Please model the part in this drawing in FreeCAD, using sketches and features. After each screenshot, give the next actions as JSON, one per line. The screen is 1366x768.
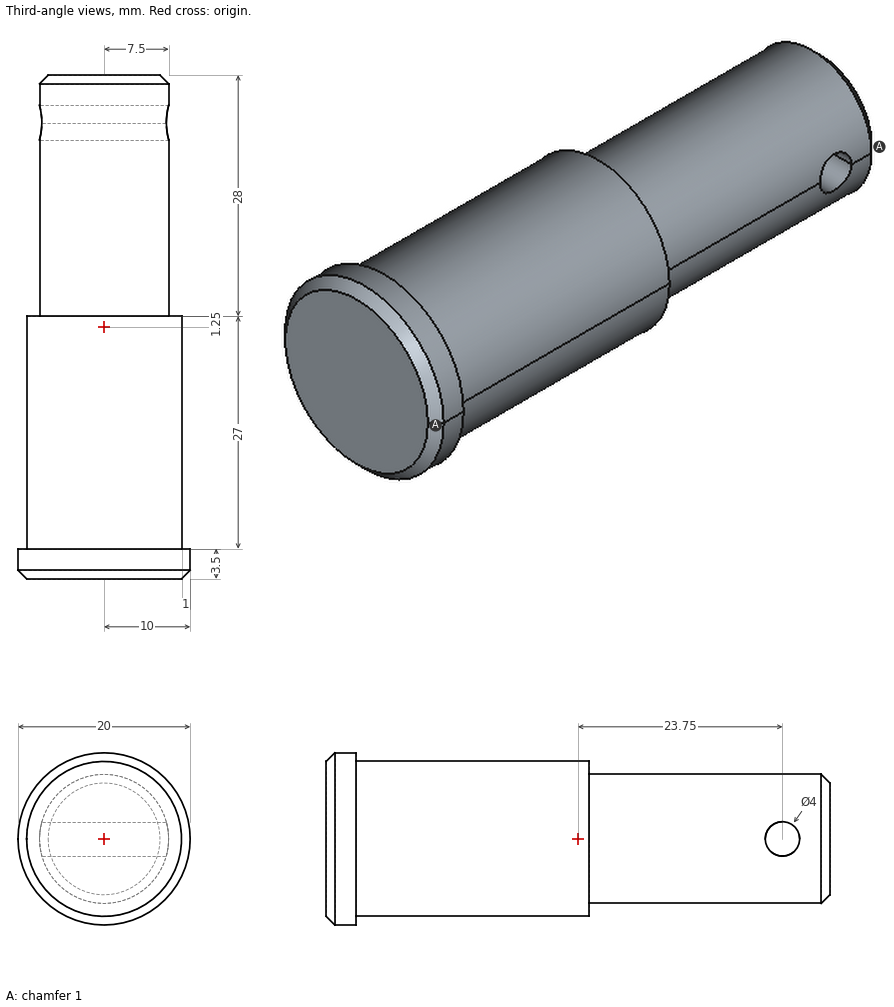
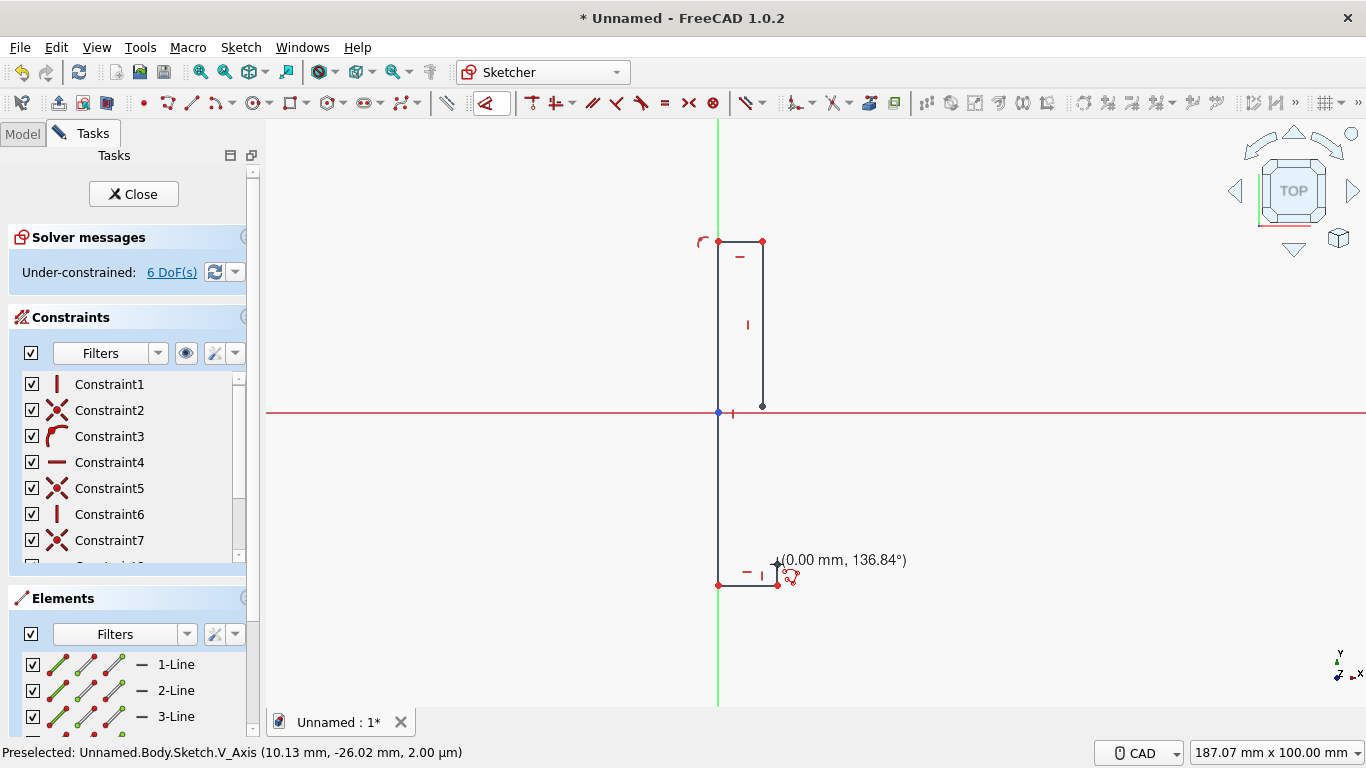
{"action": "scroll", "coordinate": [771, 564], "scroll_direction": "up", "scroll_amount": 5}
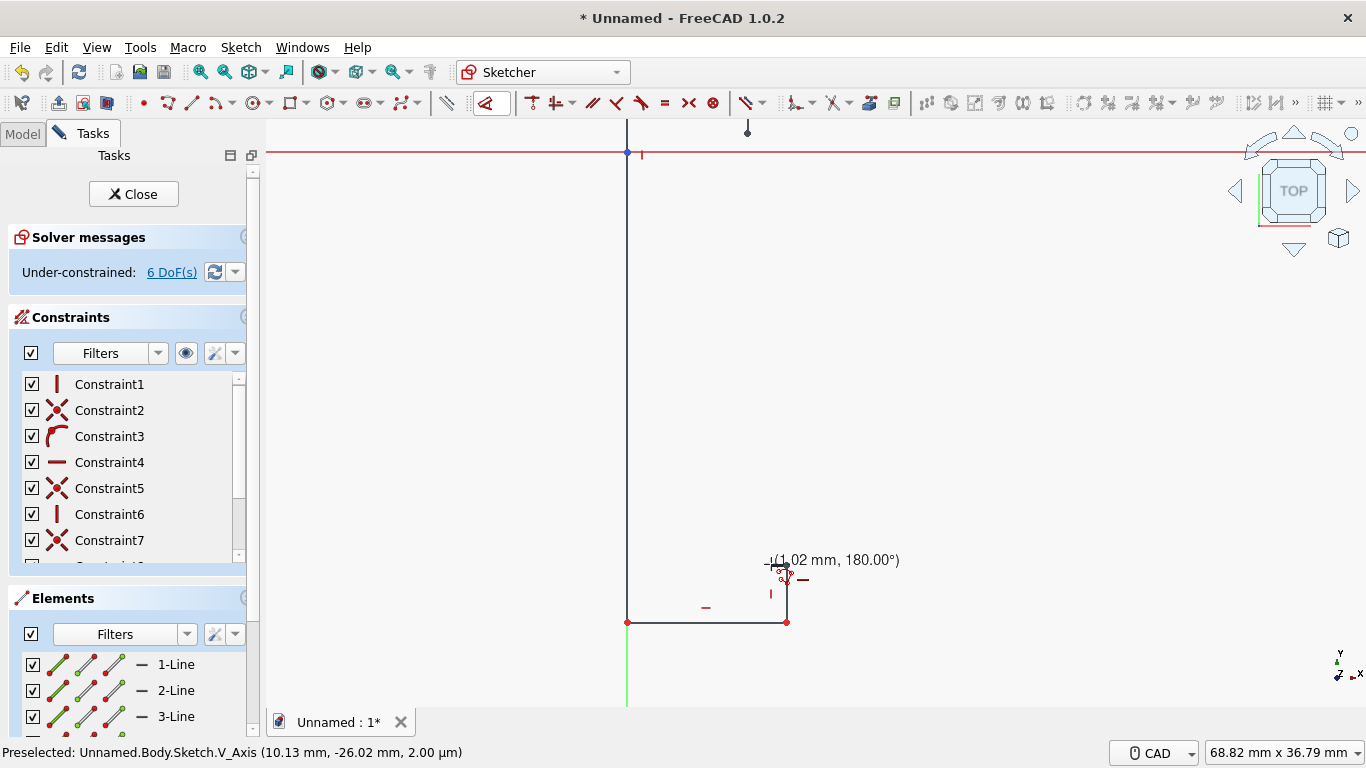
{"action": "left_click", "coordinate": [771, 563]}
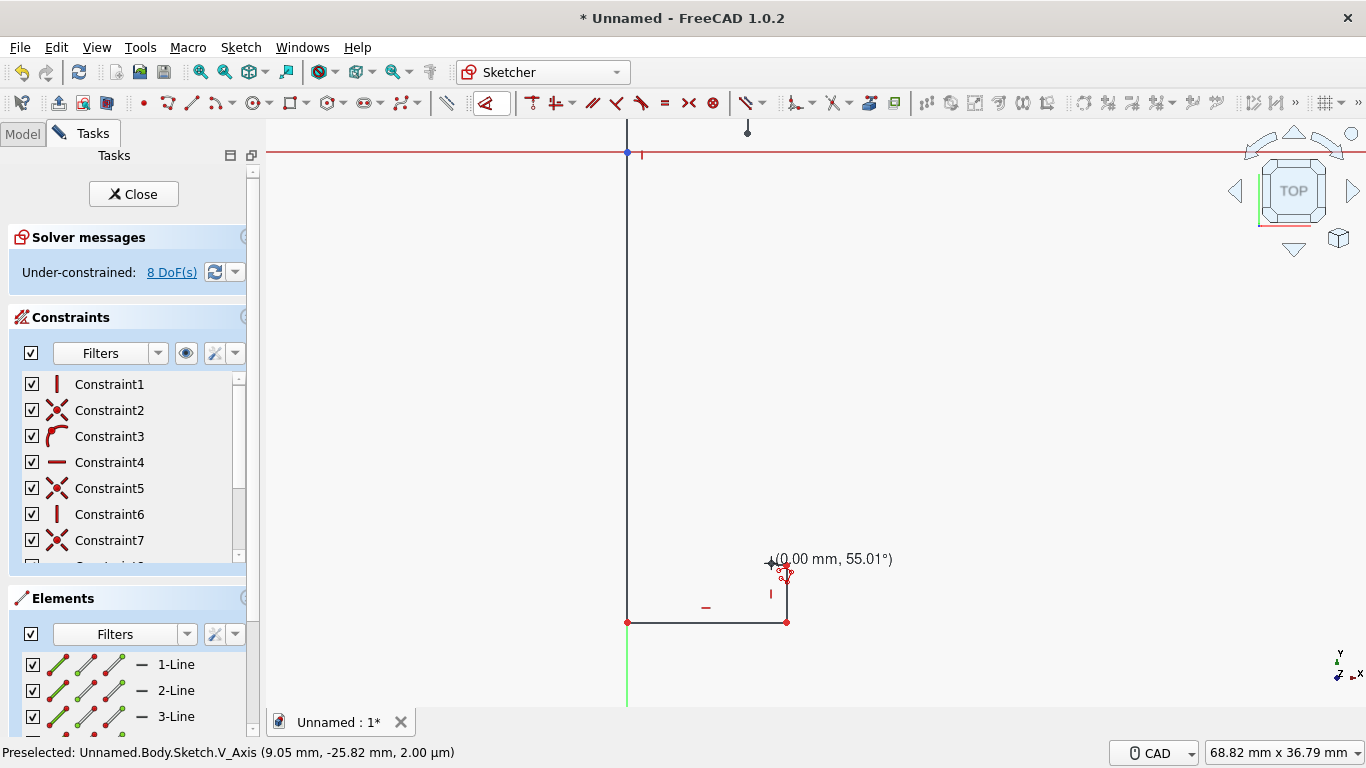
{"action": "scroll", "coordinate": [771, 565], "scroll_direction": "down", "scroll_amount": 5}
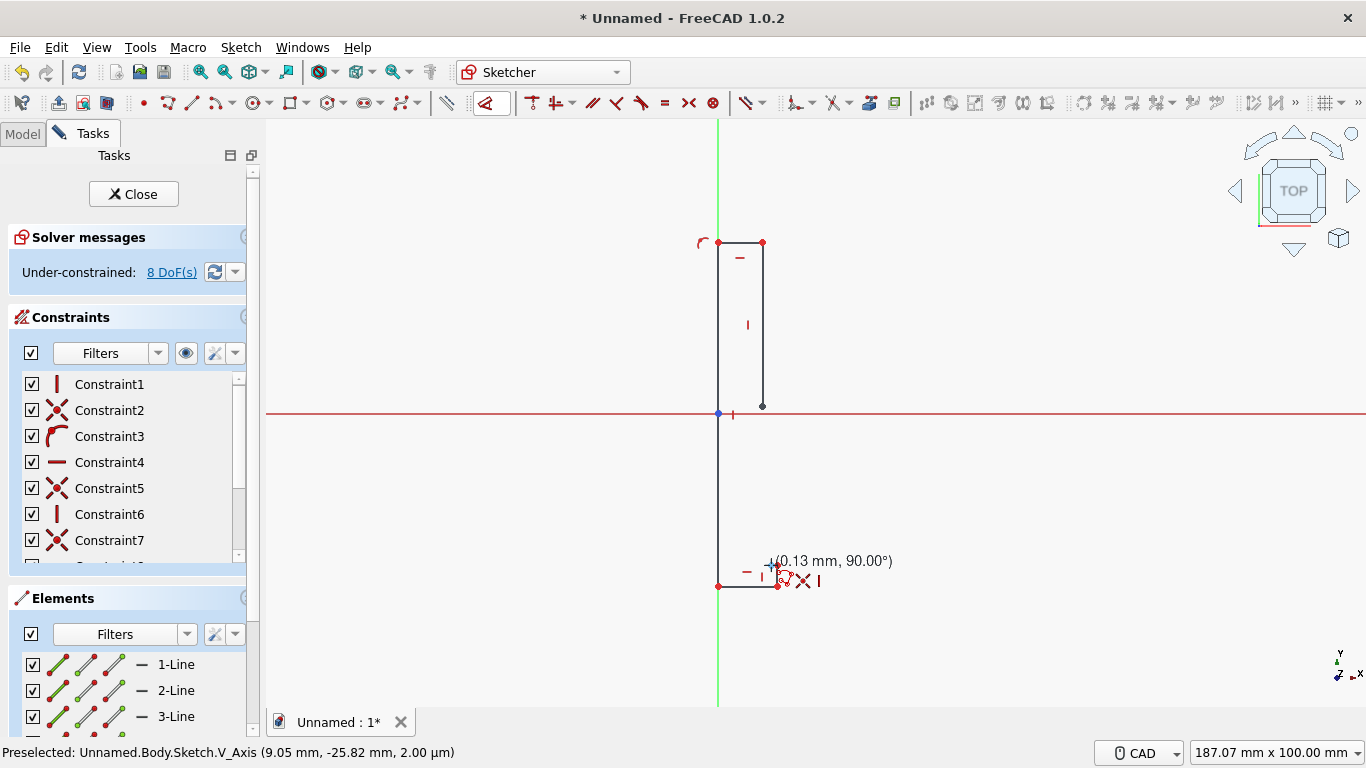
{"action": "scroll", "coordinate": [771, 406], "scroll_direction": "up", "scroll_amount": 4}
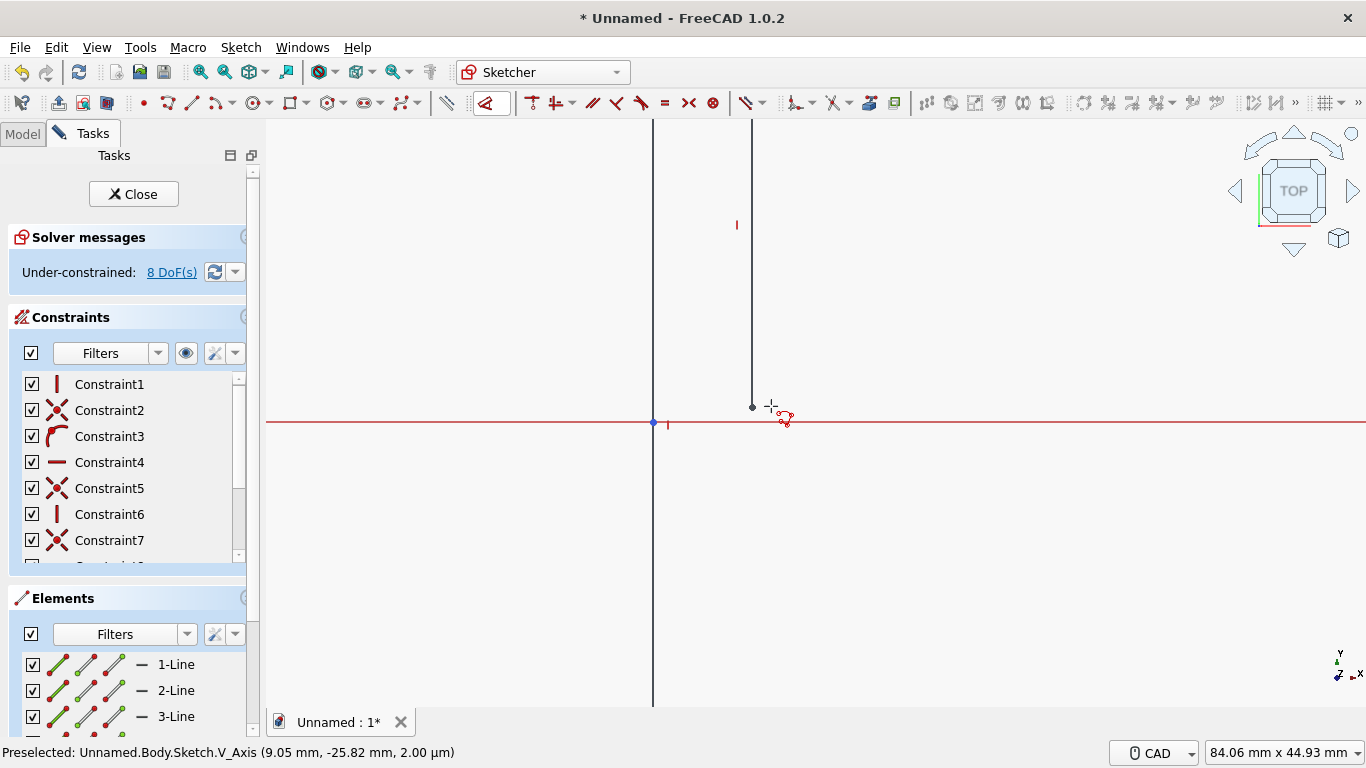
{"action": "left_click", "coordinate": [771, 406]}
{"action": "left_click", "coordinate": [752, 407]}
{"action": "key", "text": "Escape"}
{"action": "key", "text": "Escape"}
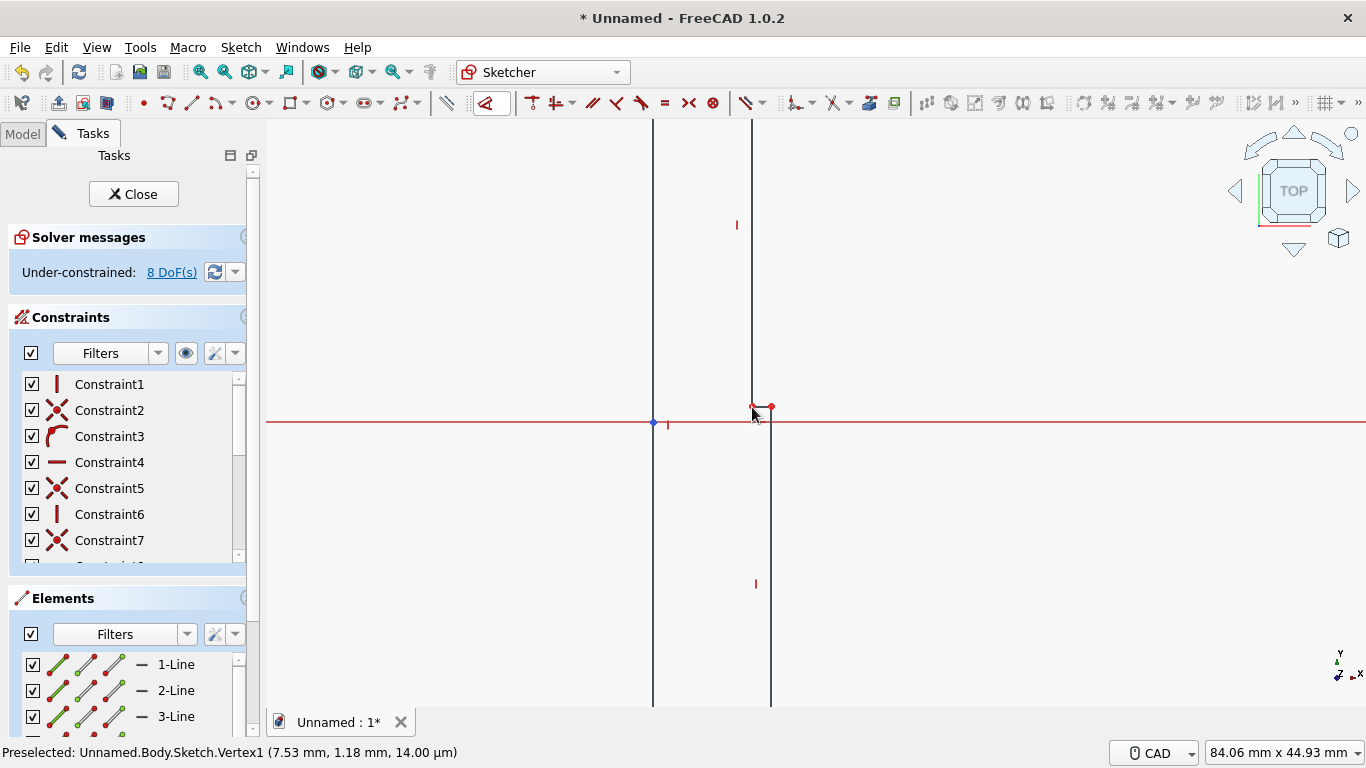
{"action": "scroll", "coordinate": [771, 405], "scroll_direction": "down", "scroll_amount": 4}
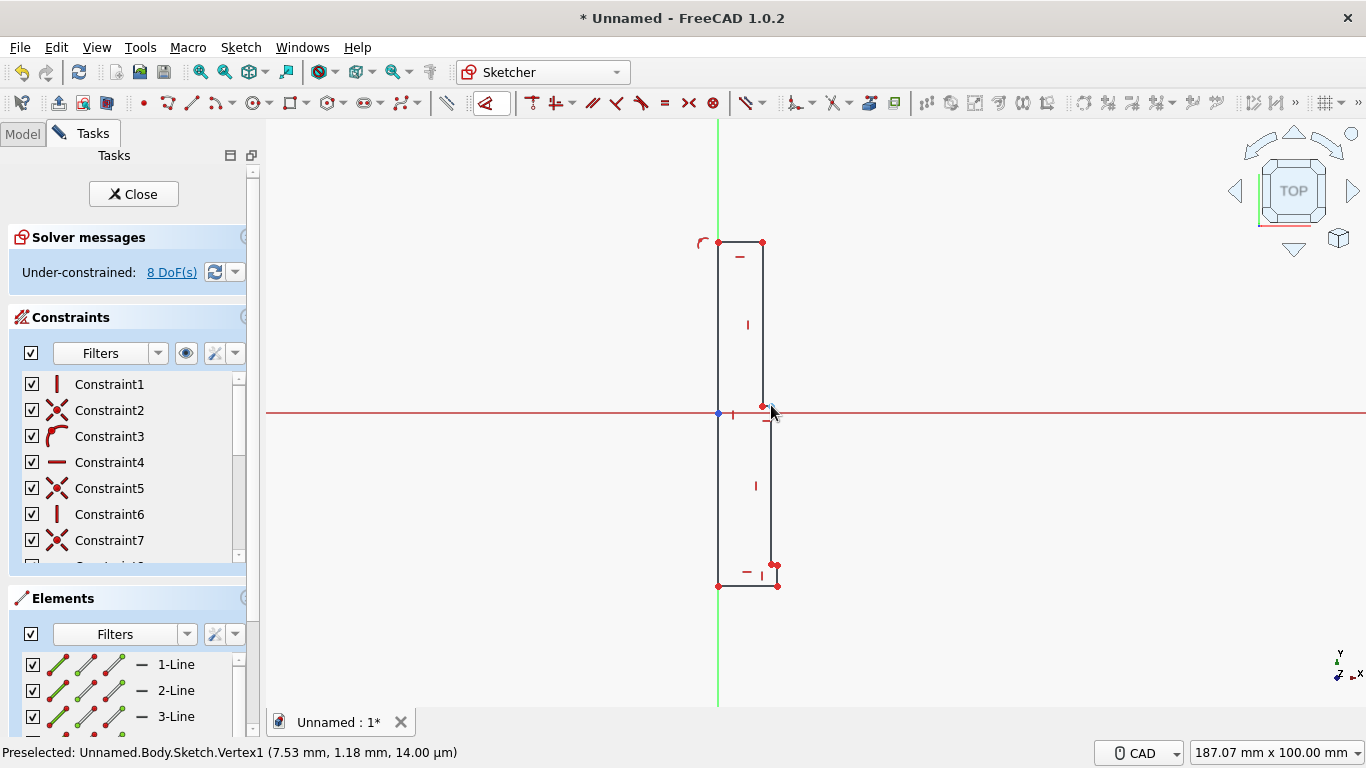
{"action": "scroll", "coordinate": [774, 565], "scroll_direction": "up", "scroll_amount": 8}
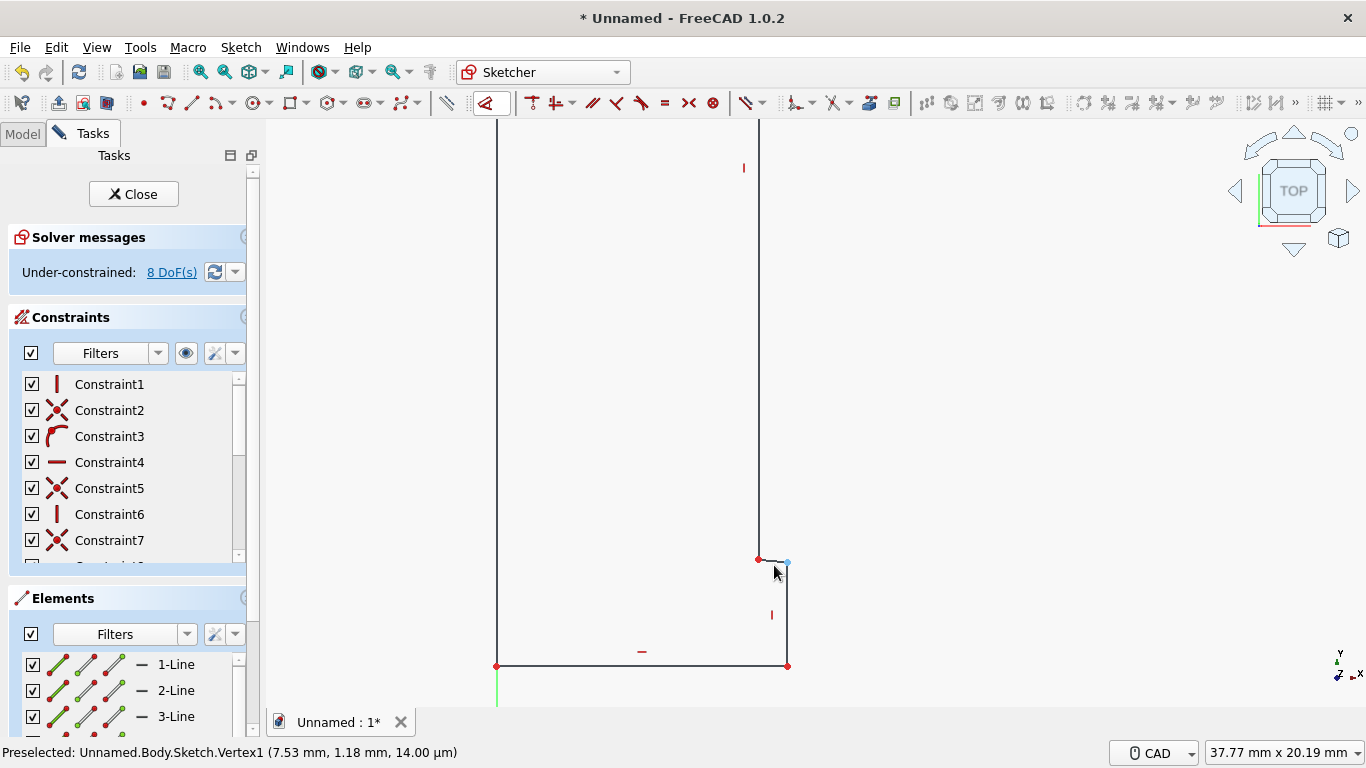
{"action": "left_click", "coordinate": [773, 561]}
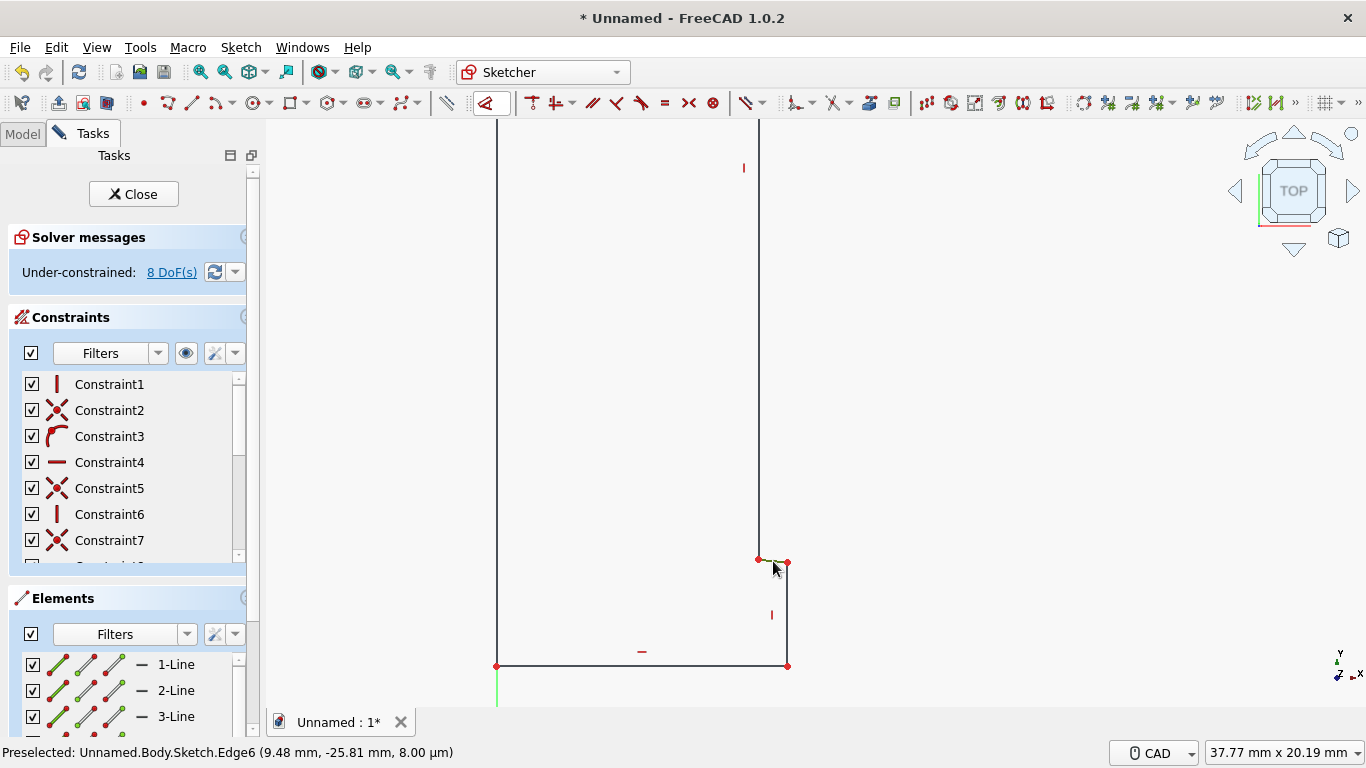
{"action": "key", "text": "h"}